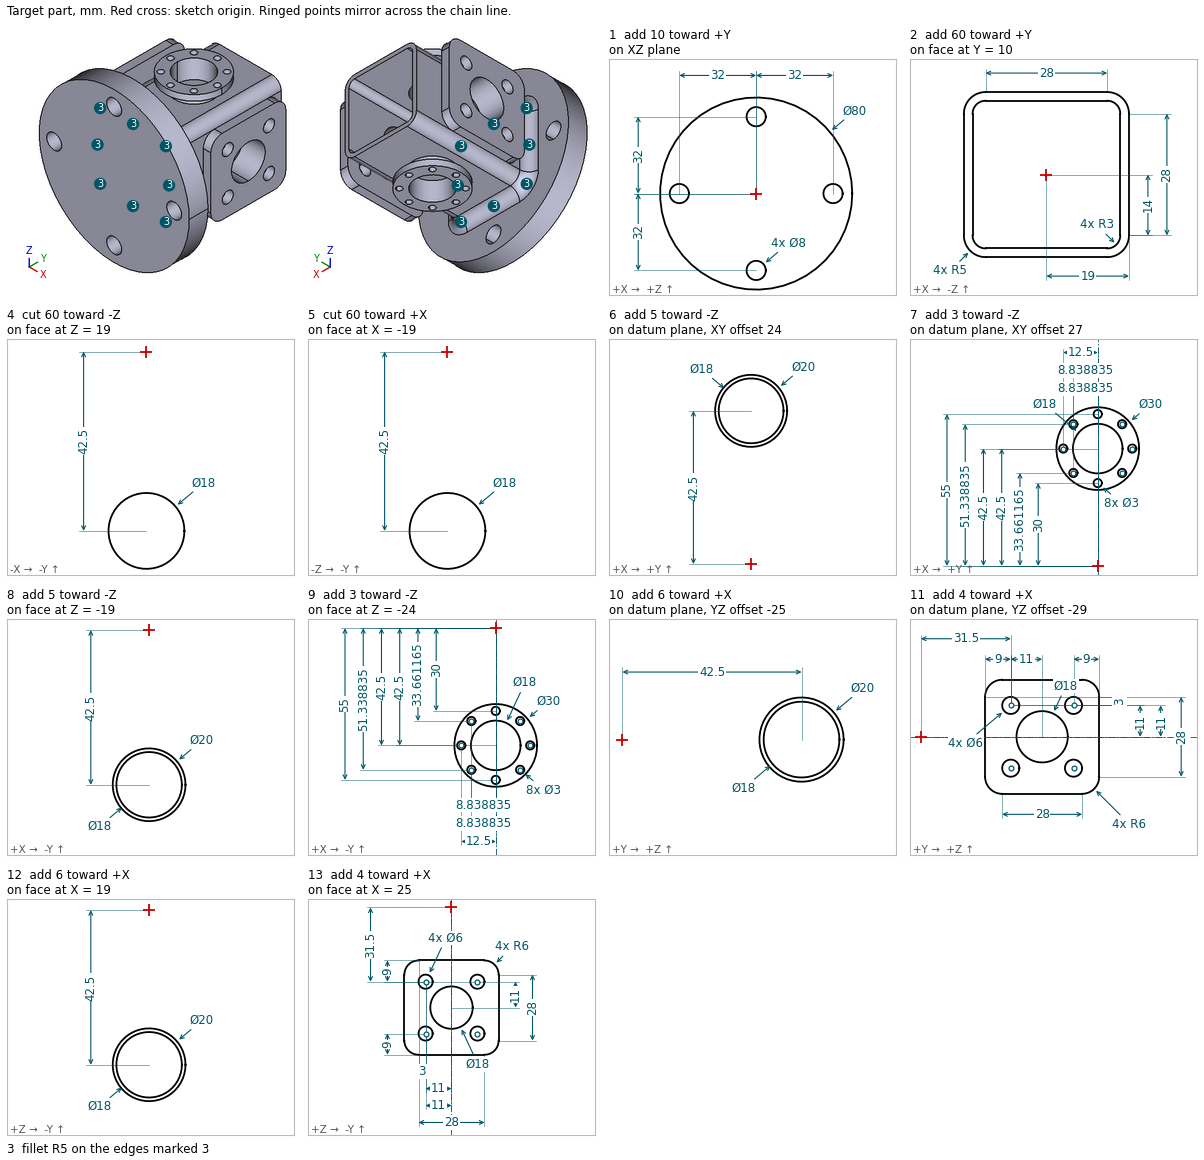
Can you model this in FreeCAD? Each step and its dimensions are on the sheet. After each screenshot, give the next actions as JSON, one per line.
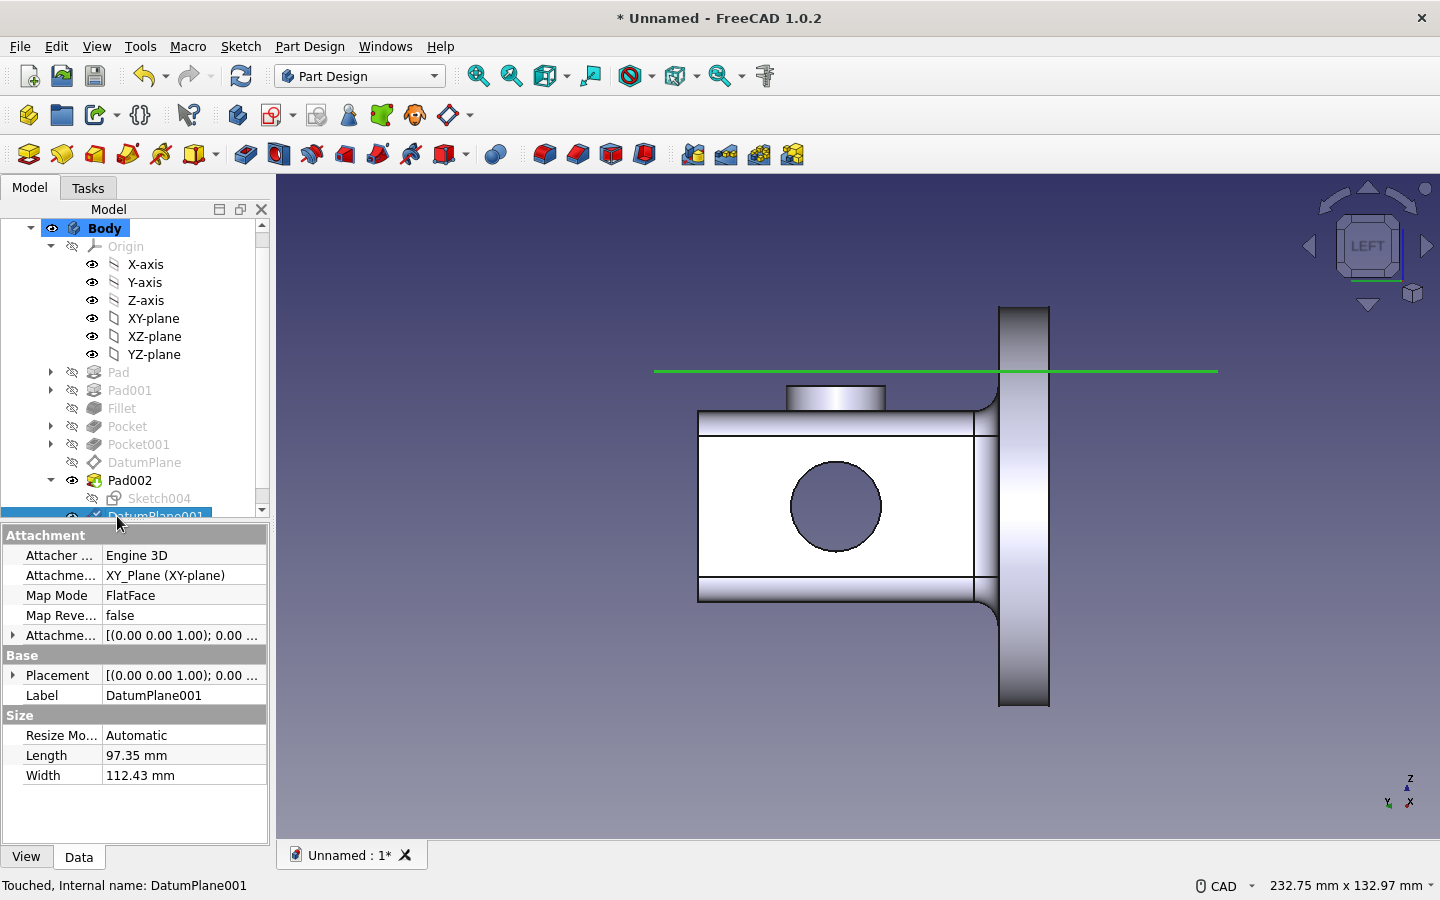
{"action": "left_click", "coordinate": [270, 116]}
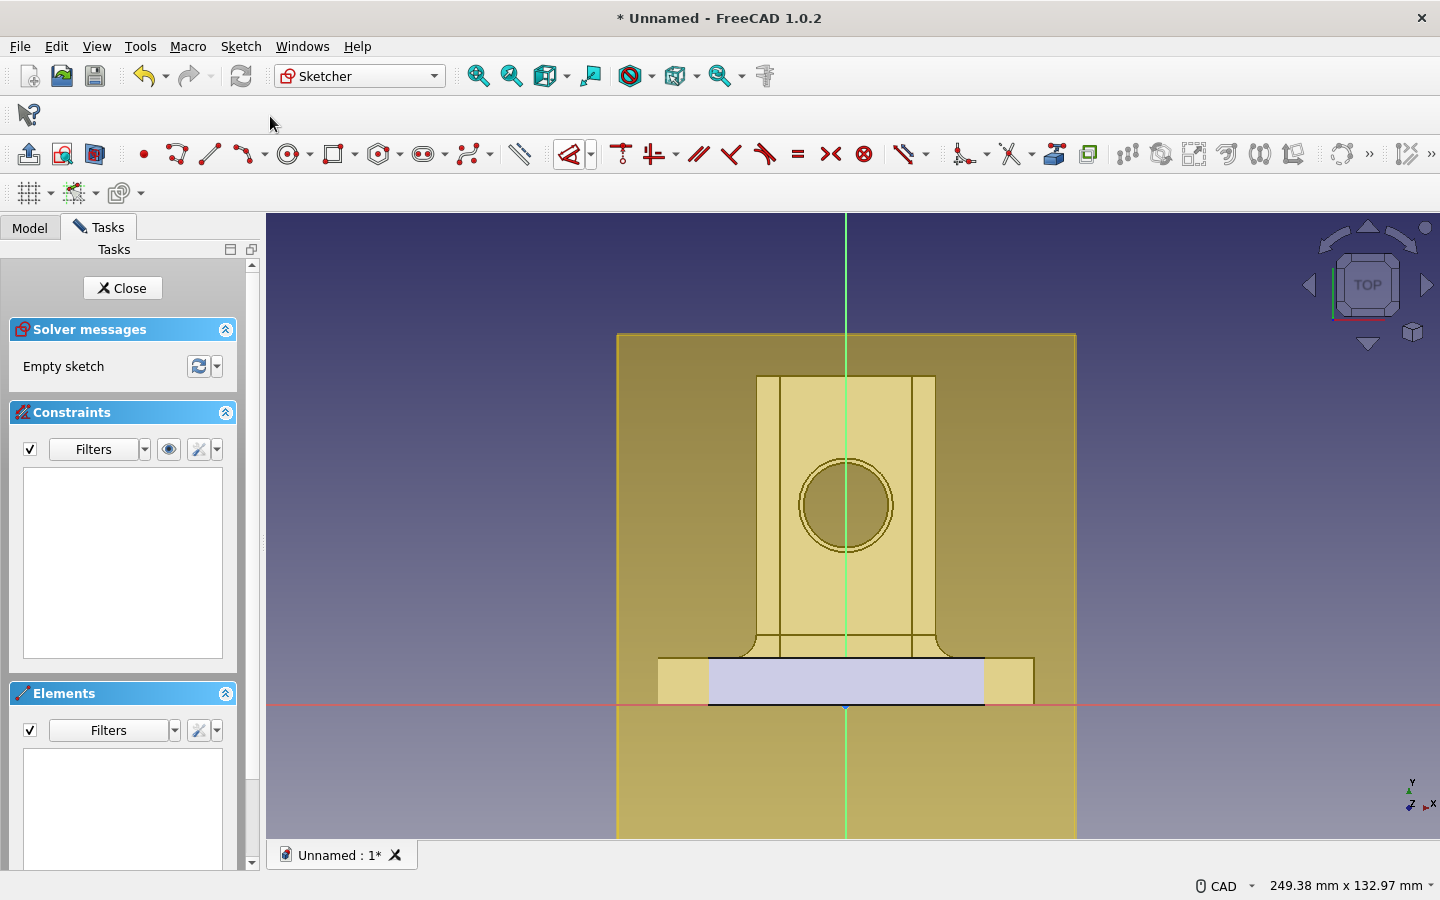
{"action": "key", "text": "q s"}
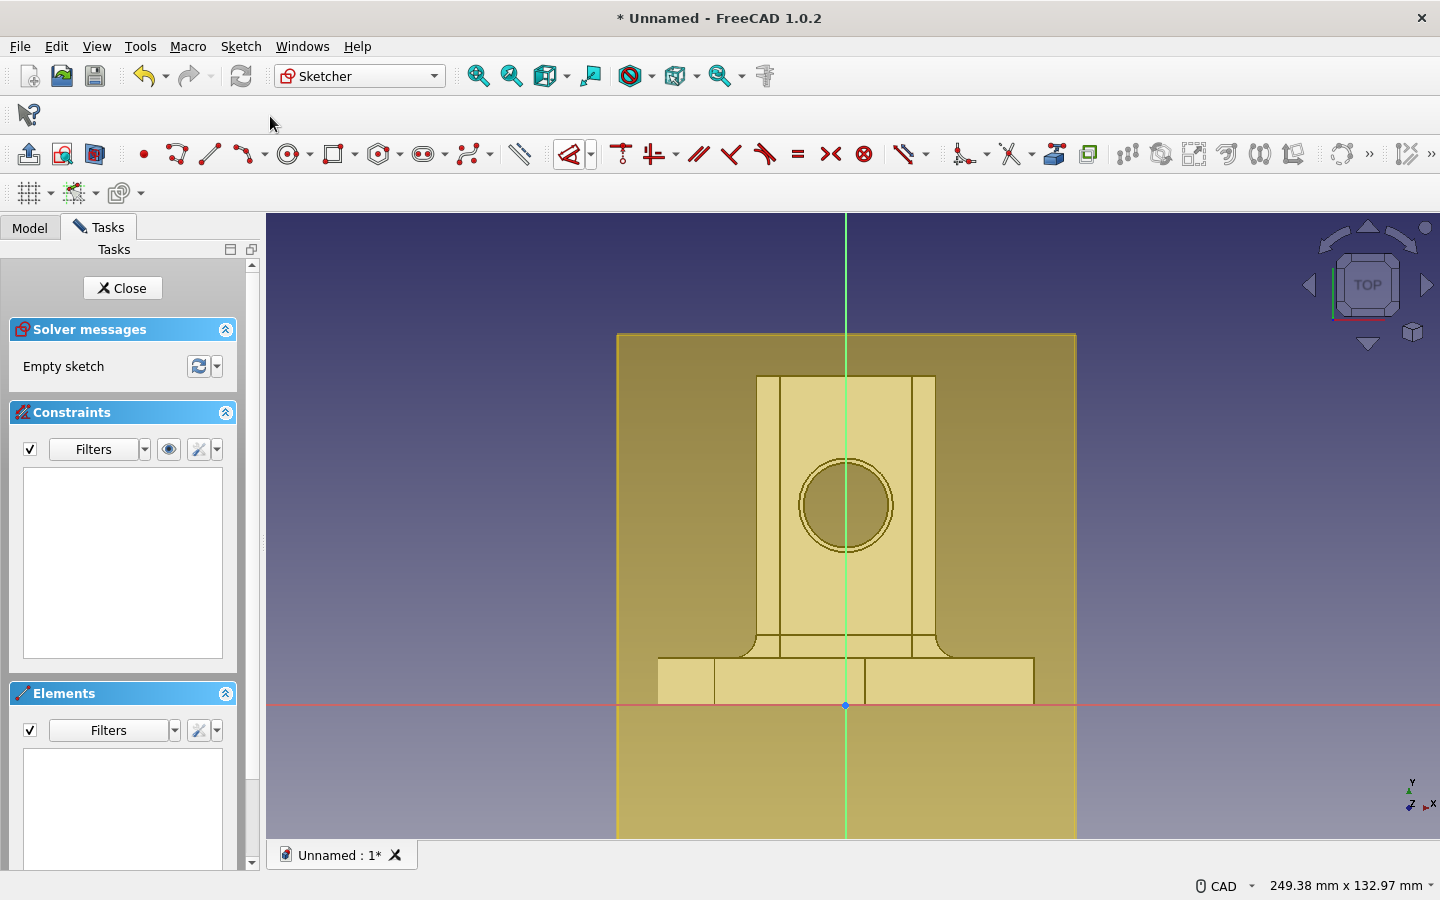
{"action": "scroll", "coordinate": [971, 660], "scroll_direction": "up", "scroll_amount": 2}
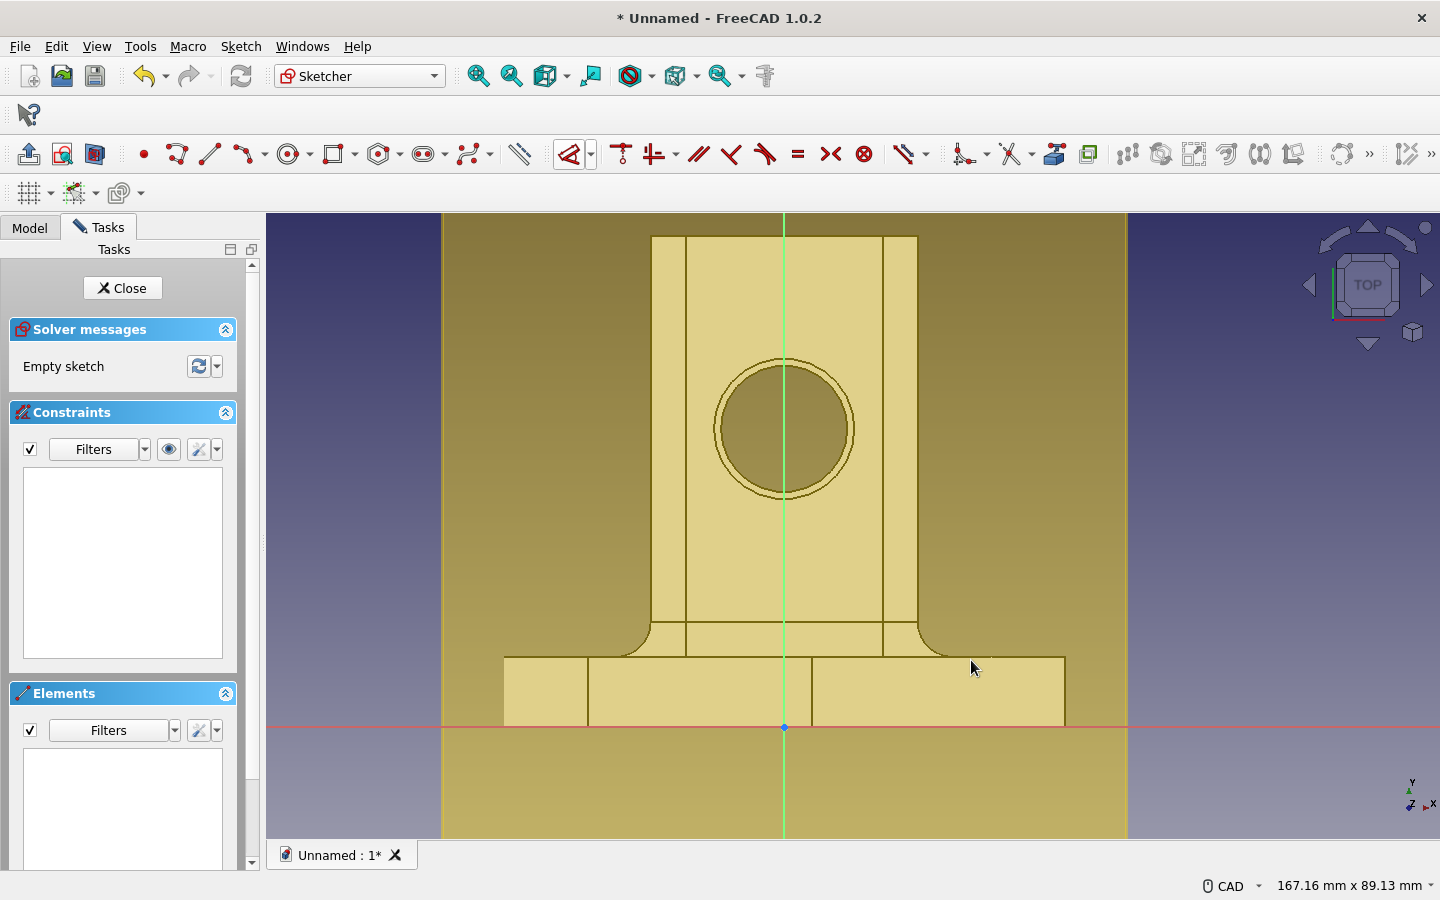
{"action": "left_click", "coordinate": [288, 154]}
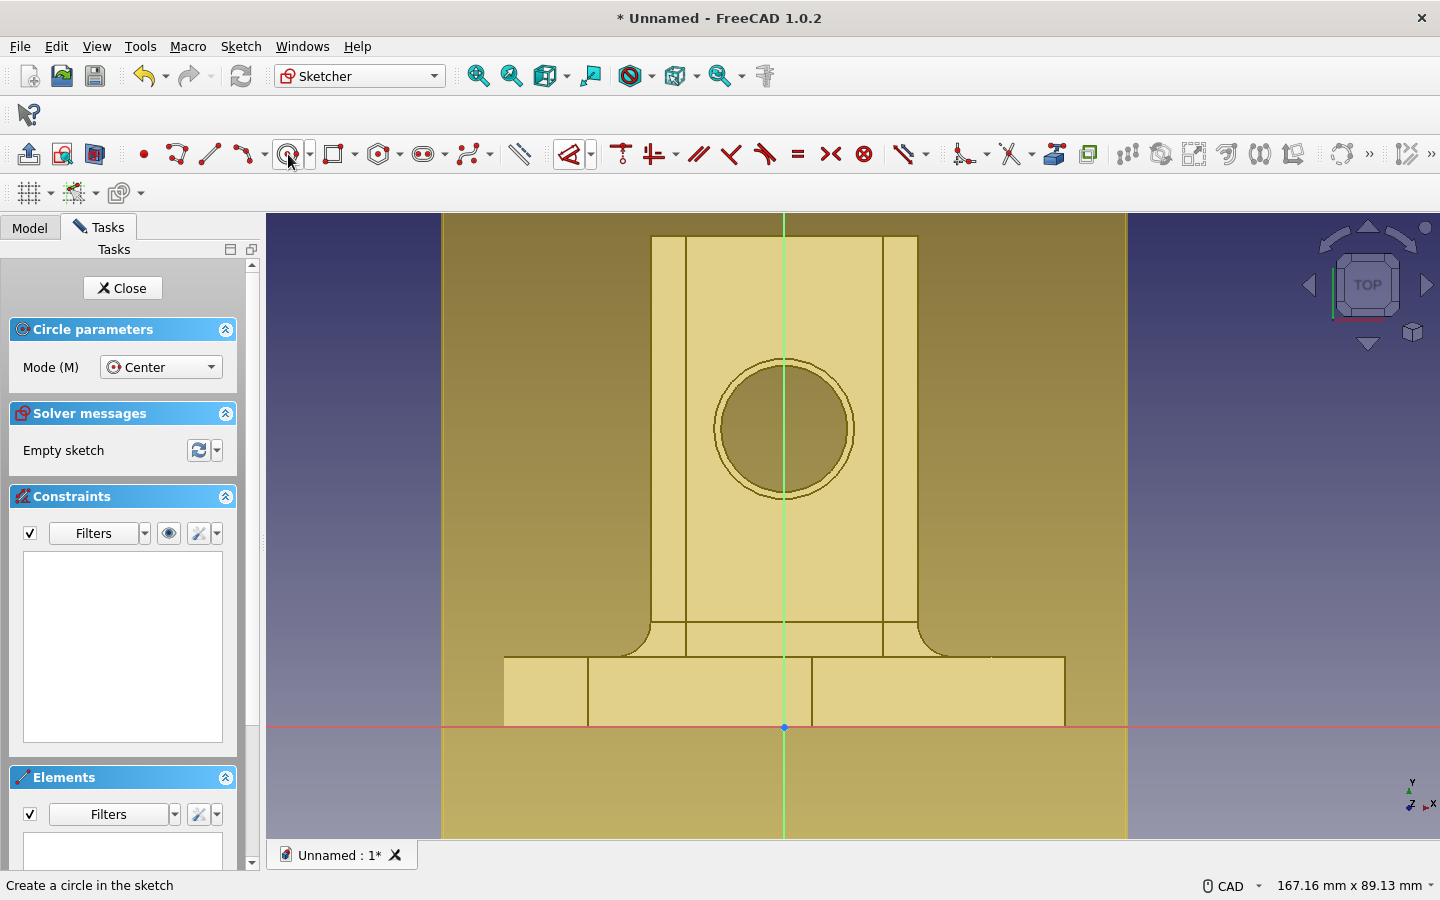
{"action": "left_click", "coordinate": [784, 429]}
{"action": "mouse_move", "coordinate": [859, 354]}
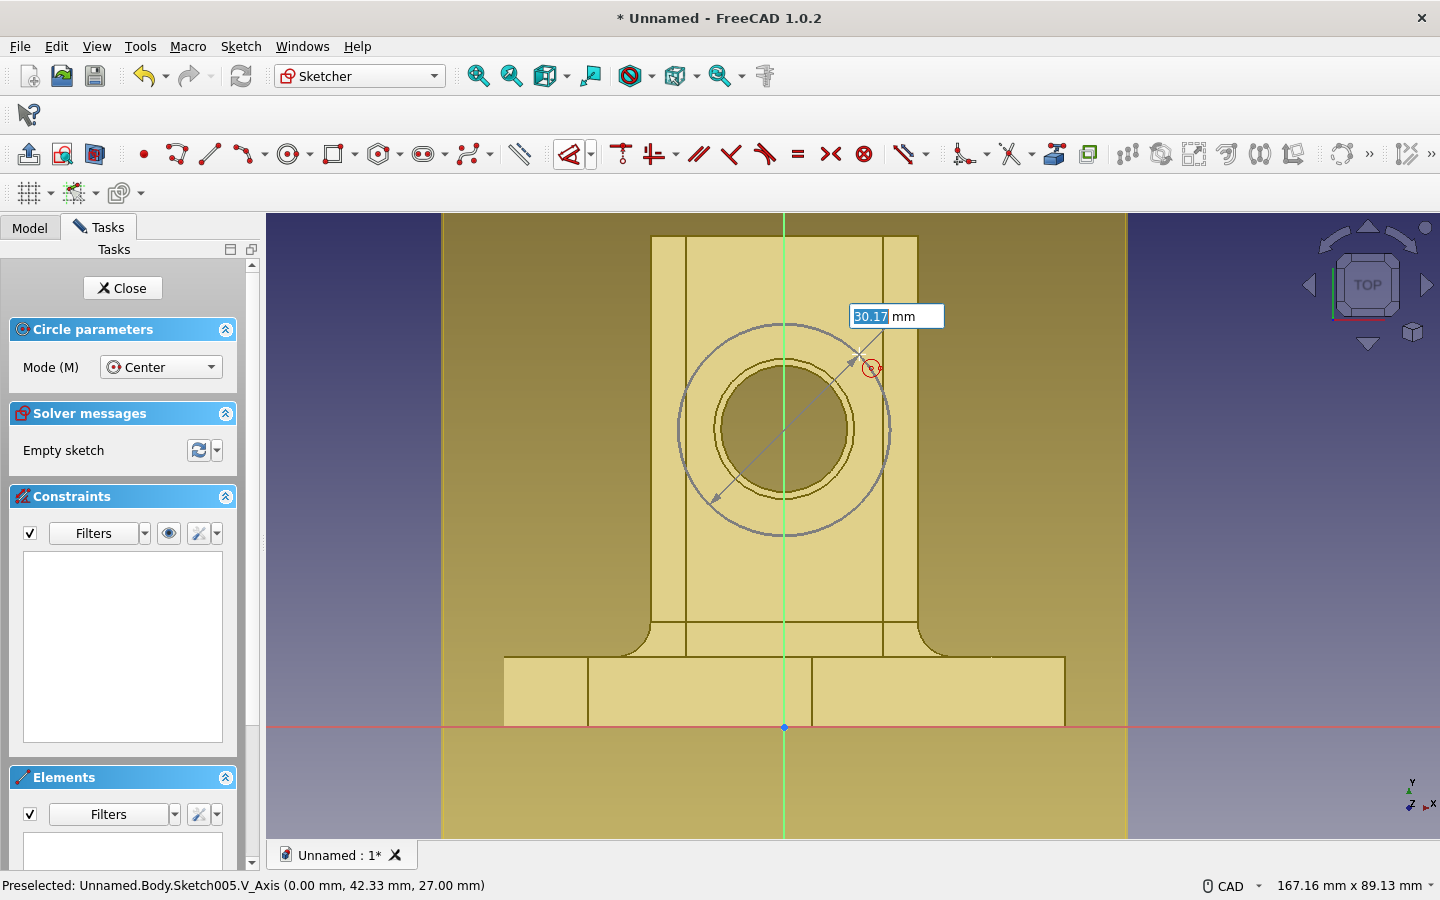
{"action": "type", "text": "30"}
{"action": "key", "text": "Return"}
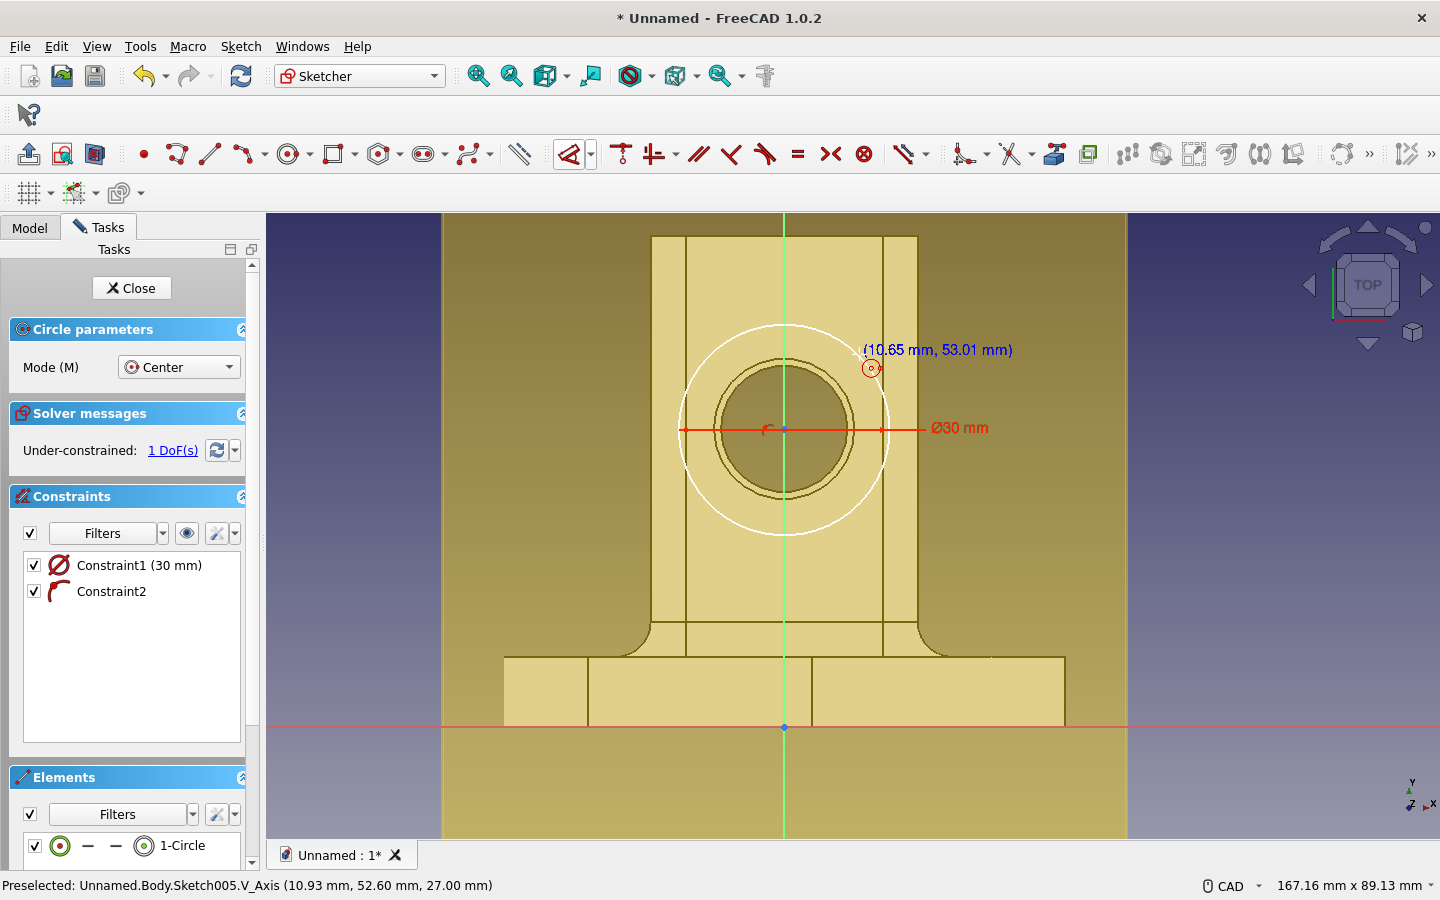
{"action": "scroll", "coordinate": [722, 491], "scroll_direction": "up", "scroll_amount": 4}